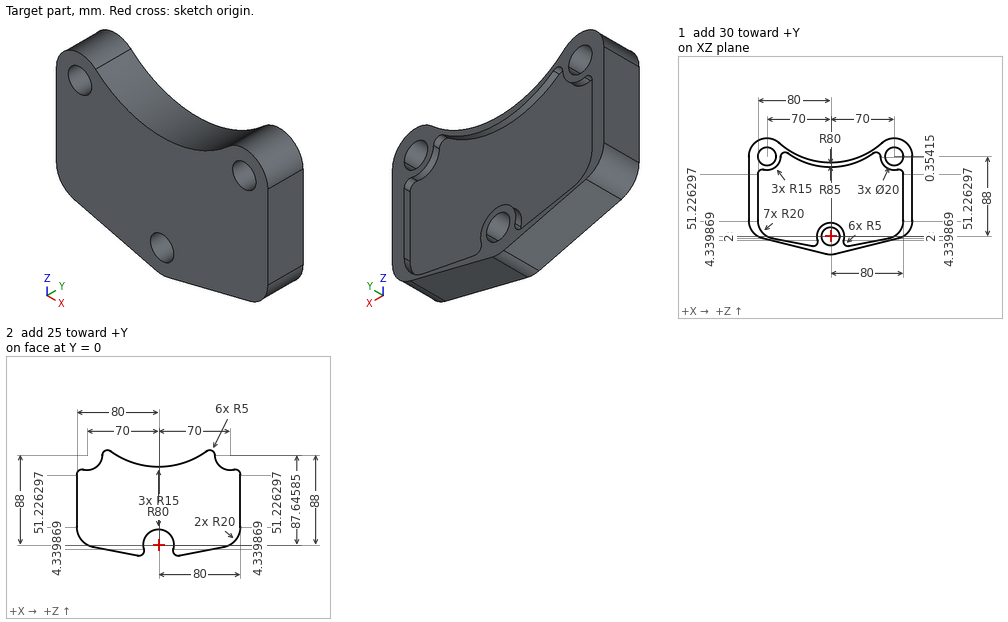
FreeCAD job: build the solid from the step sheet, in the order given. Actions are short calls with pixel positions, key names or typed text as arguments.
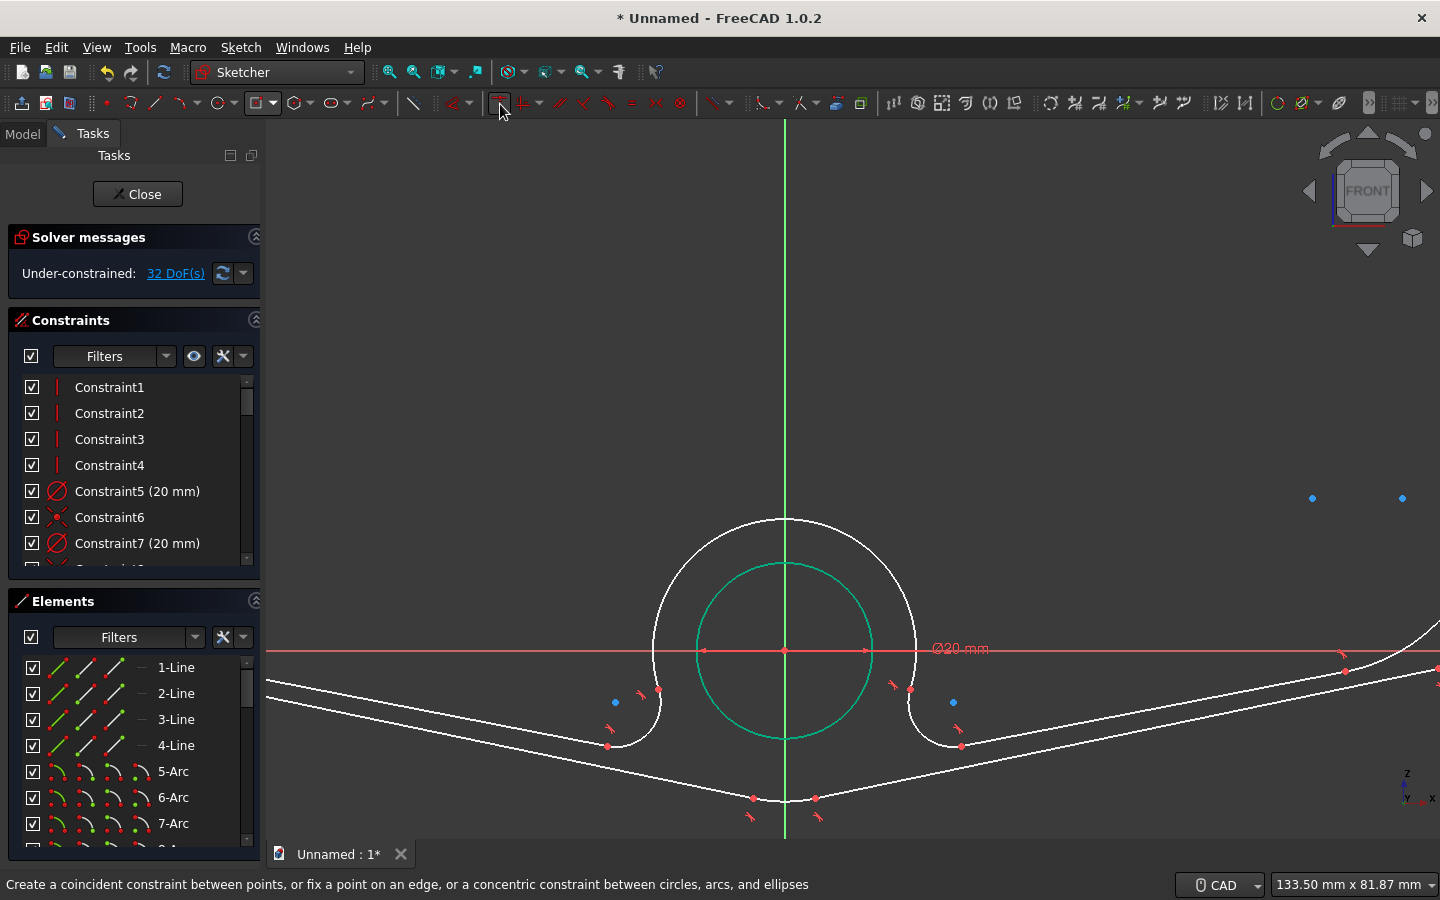
scroll(784, 648, down, 4)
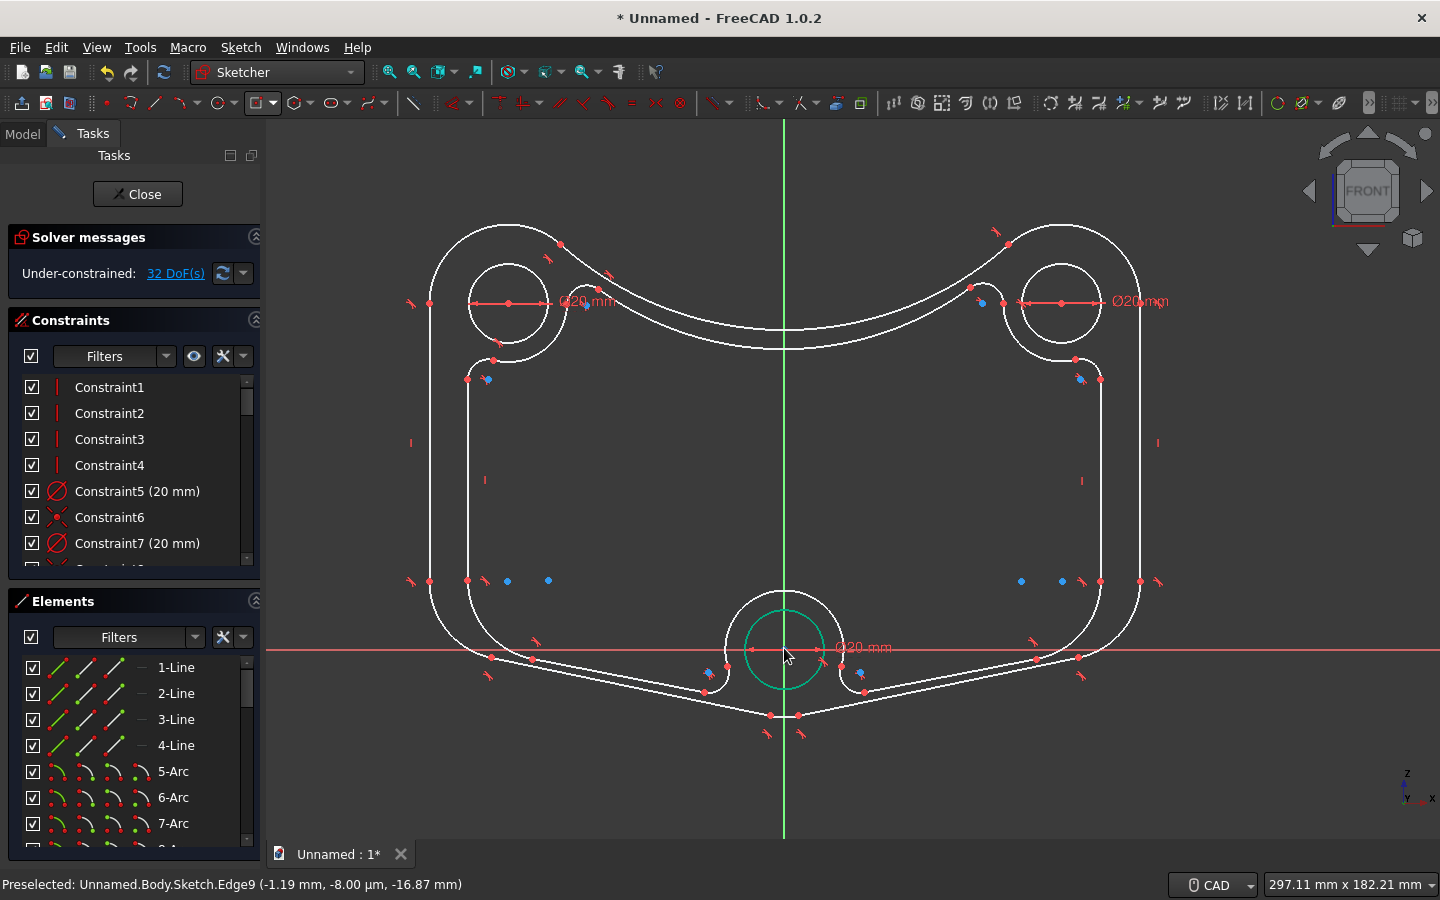
click(511, 225)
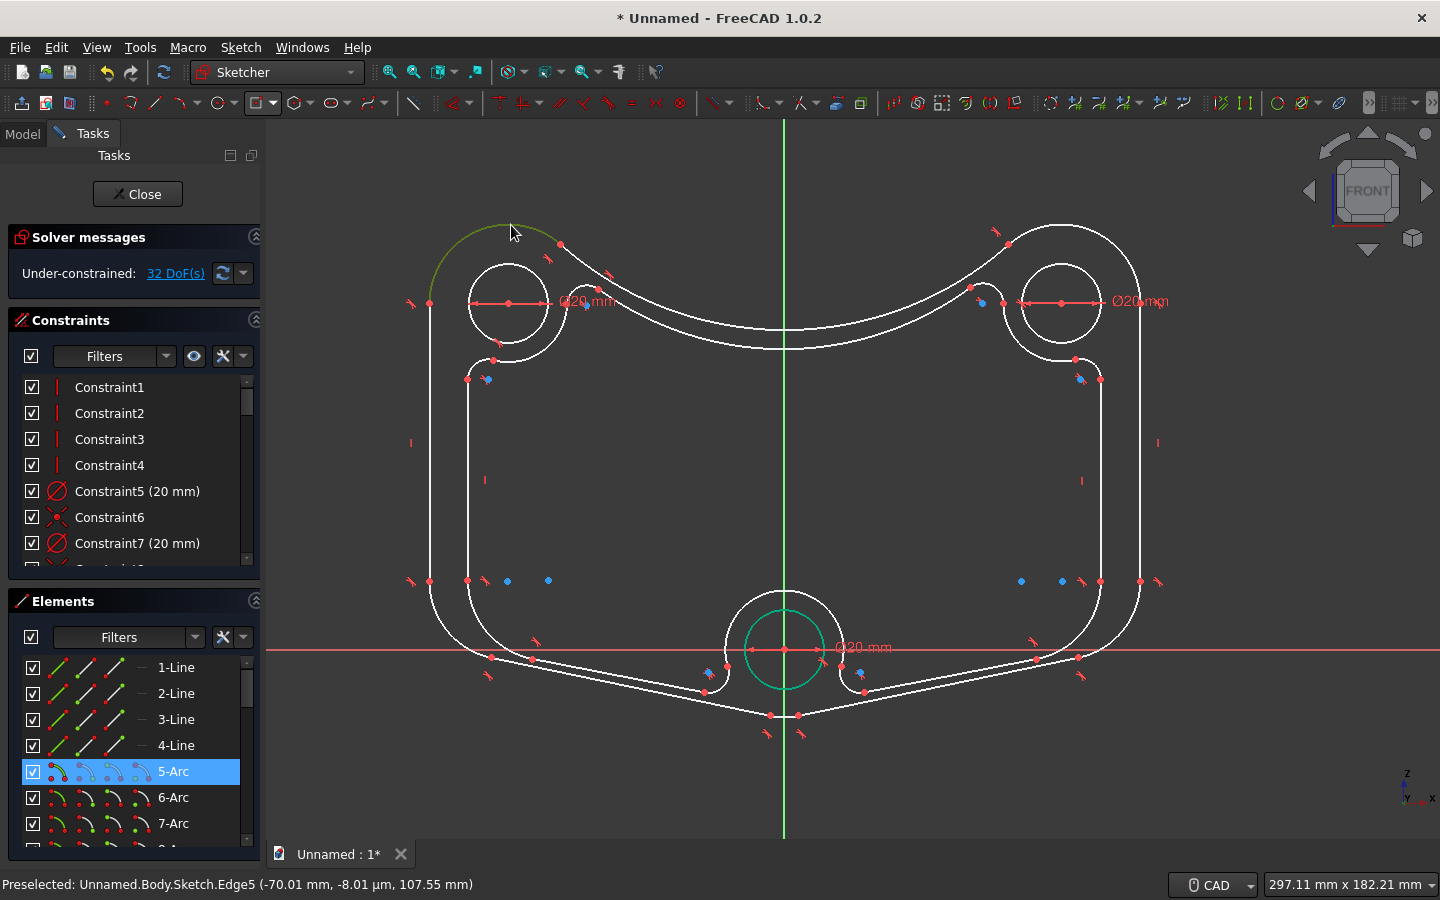
click(1122, 253)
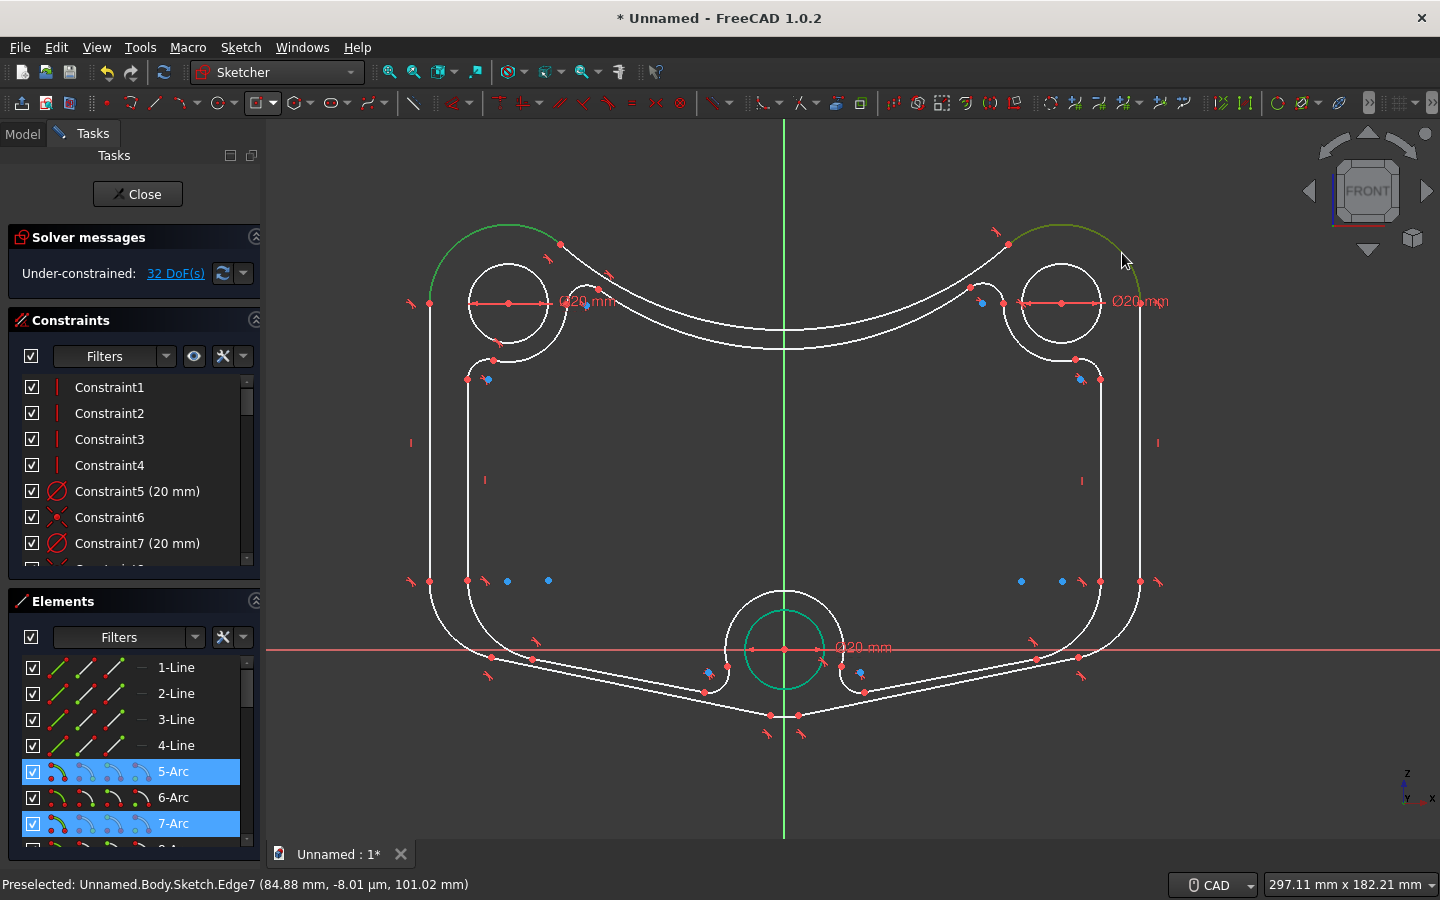
click(1134, 613)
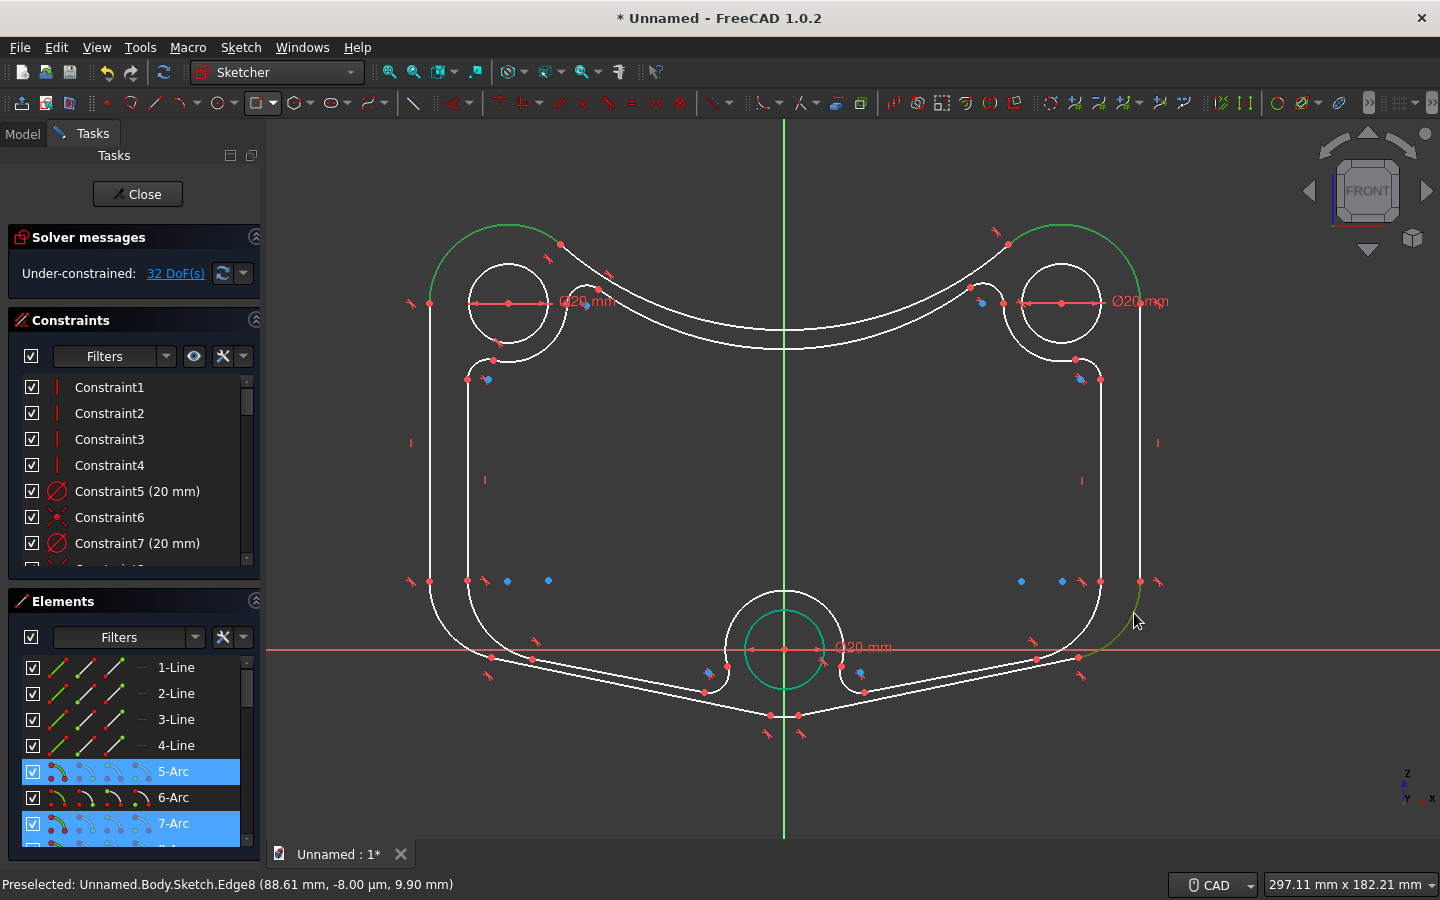
click(784, 717)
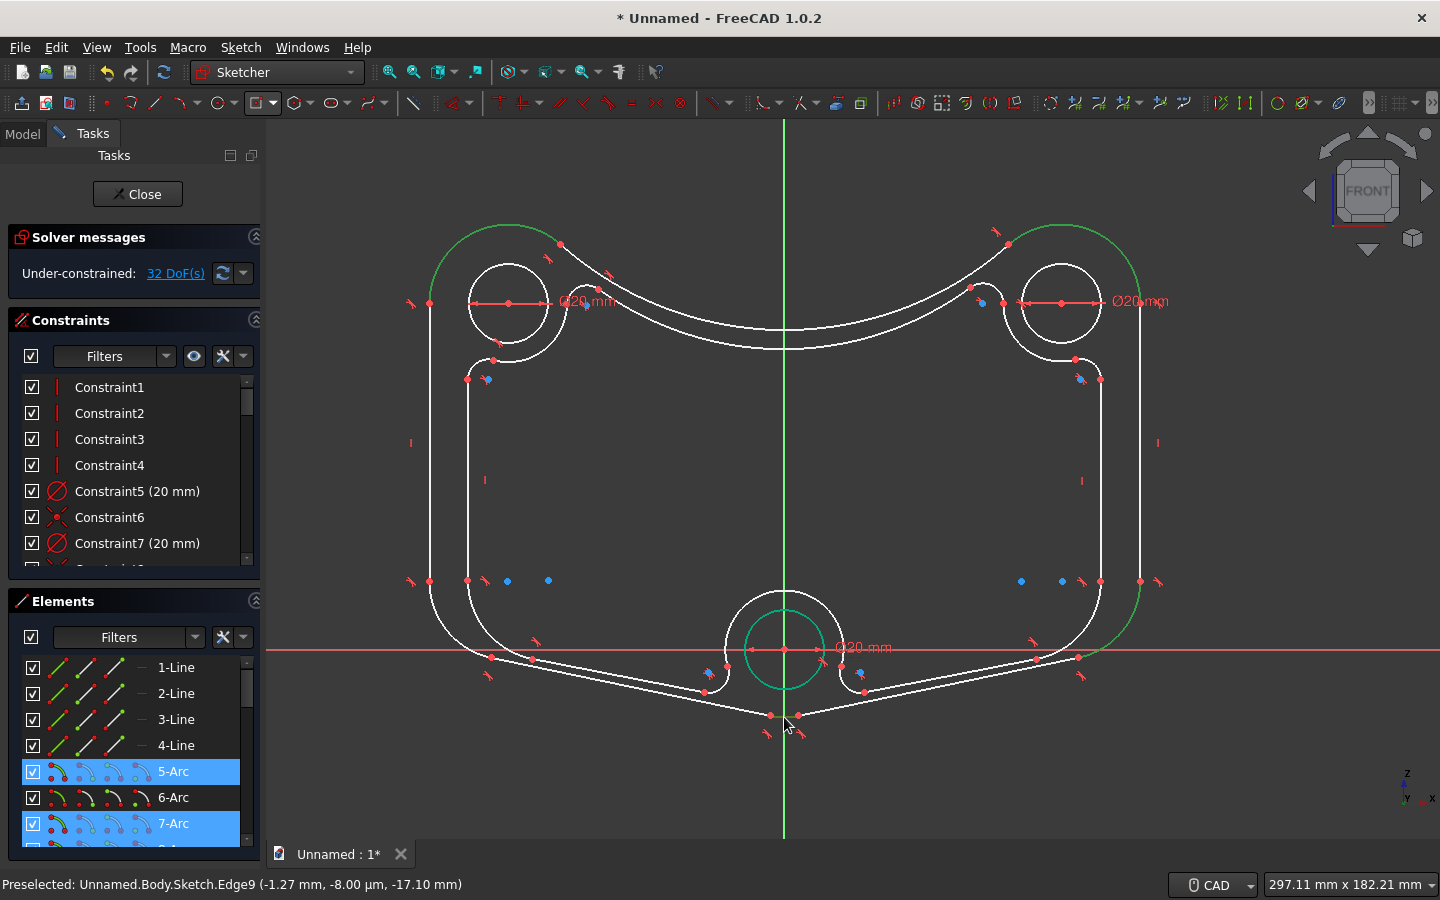
click(436, 613)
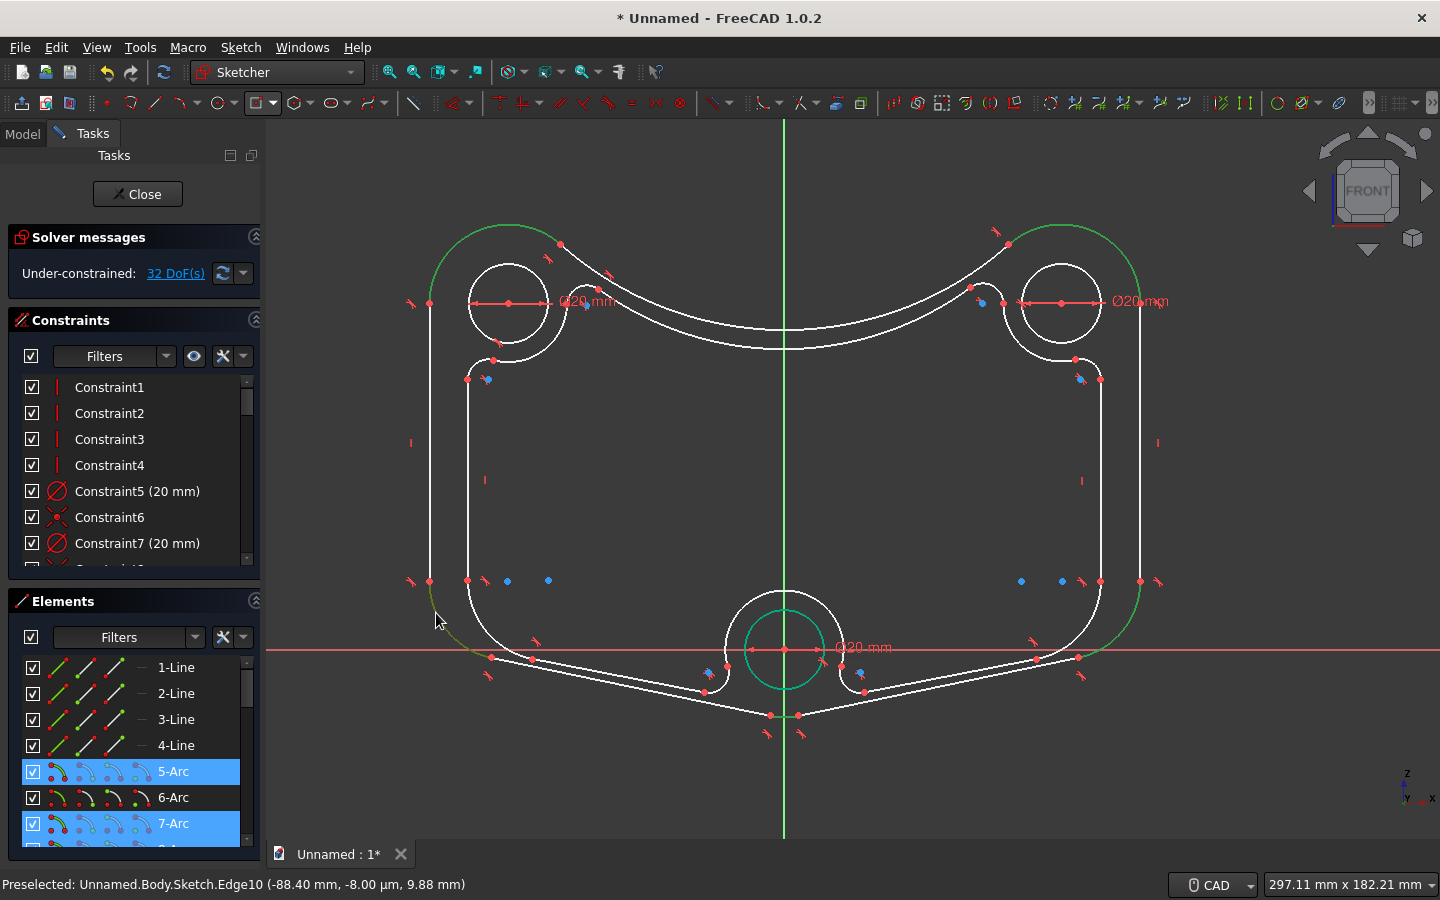
click(475, 612)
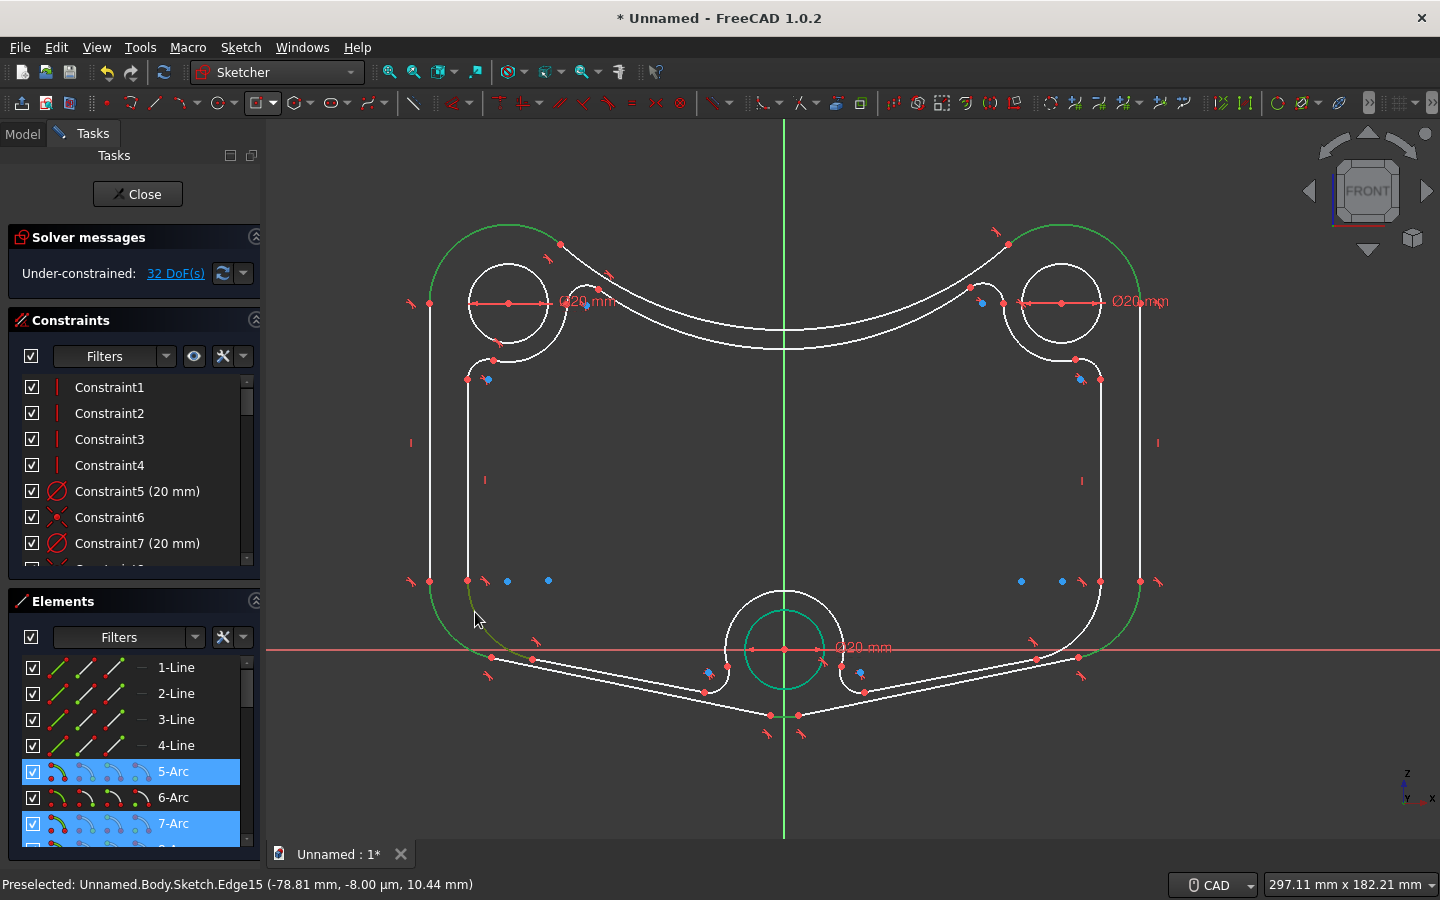
click(1067, 646)